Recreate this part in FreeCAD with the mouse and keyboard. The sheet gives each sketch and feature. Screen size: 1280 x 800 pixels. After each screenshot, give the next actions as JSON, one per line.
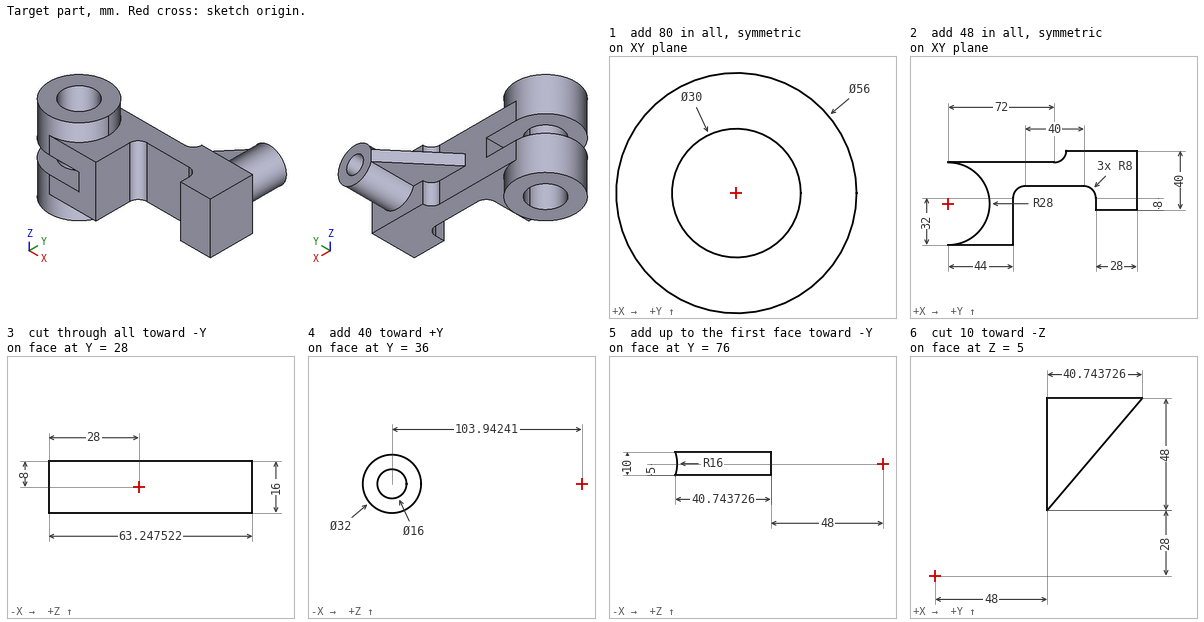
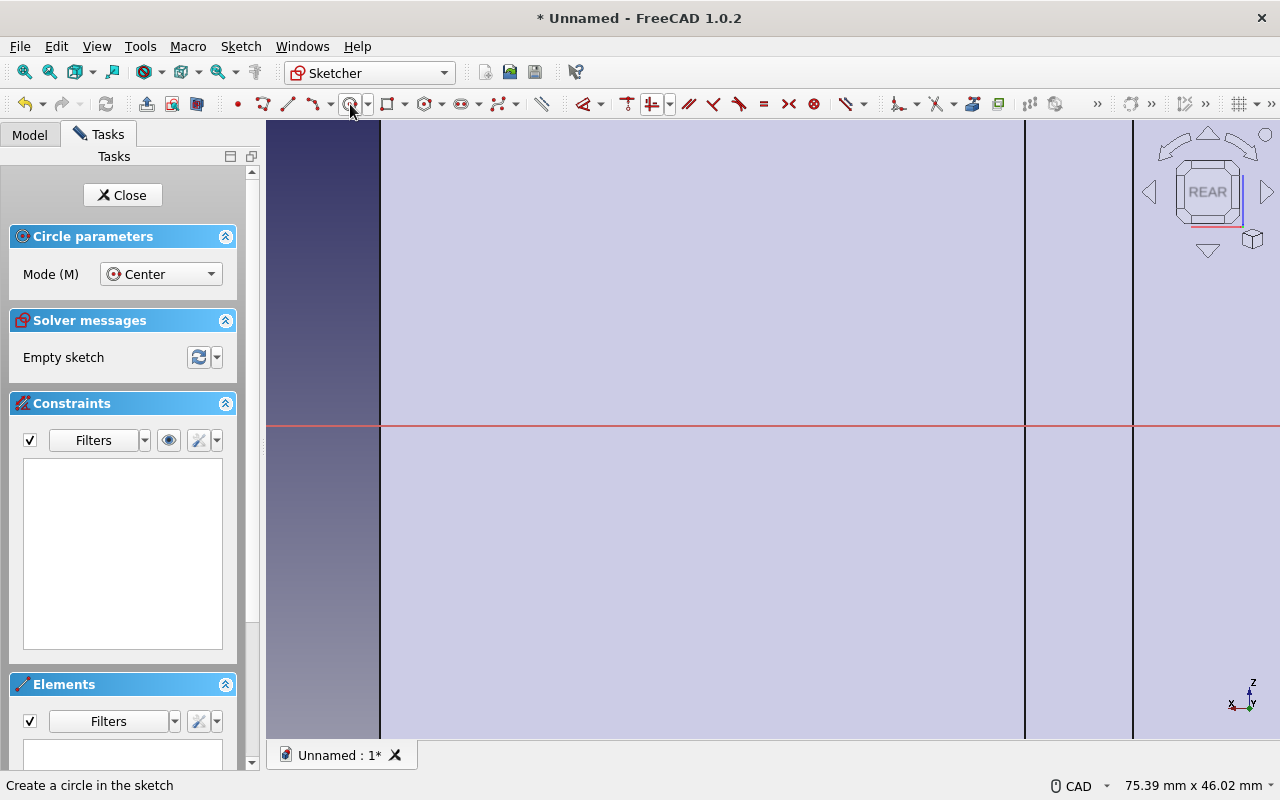
{"action": "left_click", "coordinate": [703, 426]}
{"action": "mouse_move", "coordinate": [856, 274]}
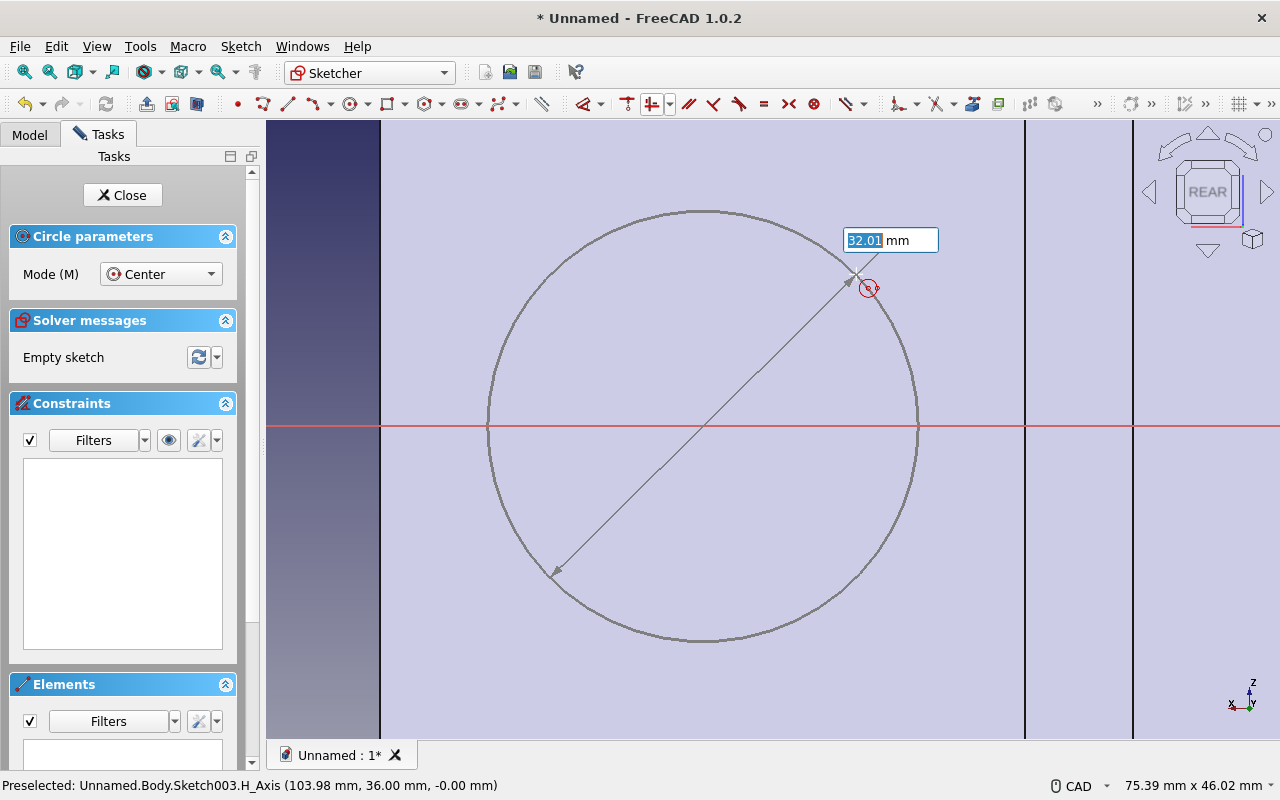
{"action": "type", "text": "32"}
{"action": "key", "text": "Return"}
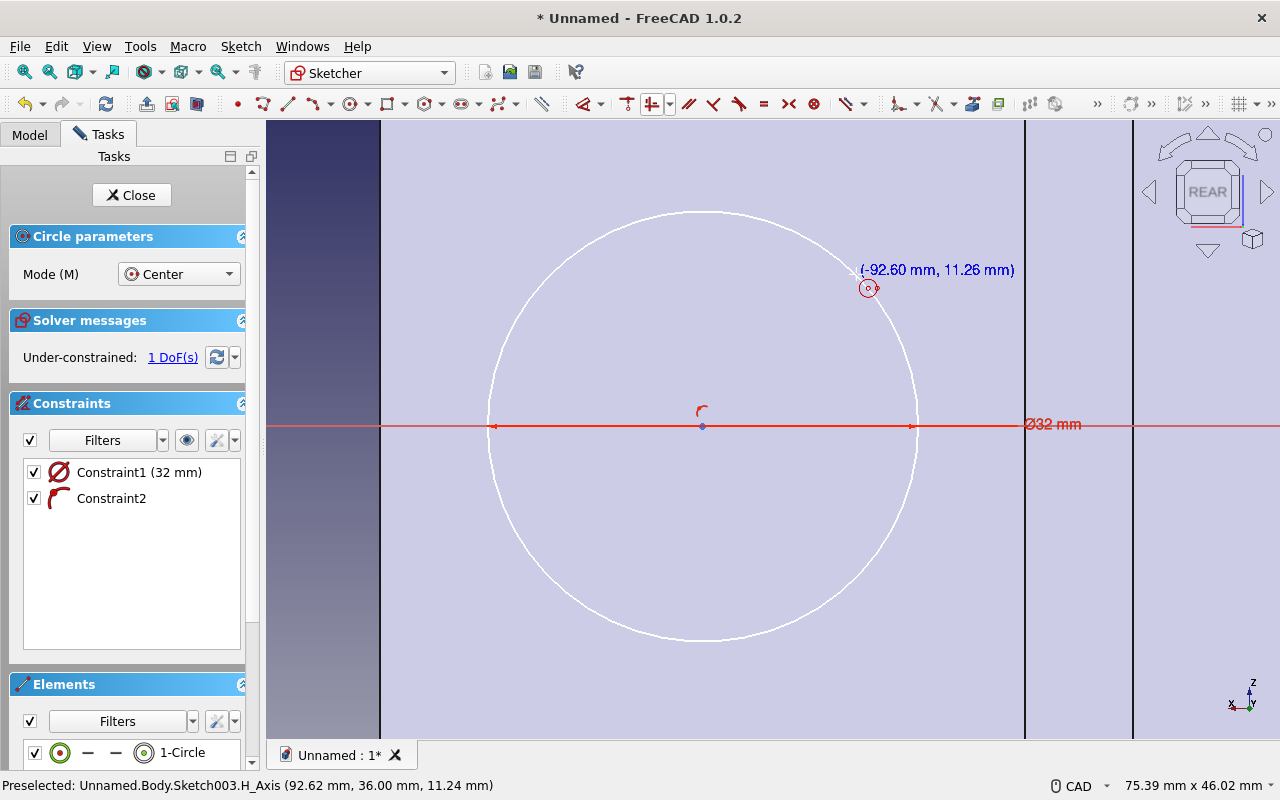
{"action": "left_click", "coordinate": [703, 426]}
{"action": "mouse_move", "coordinate": [780, 350]}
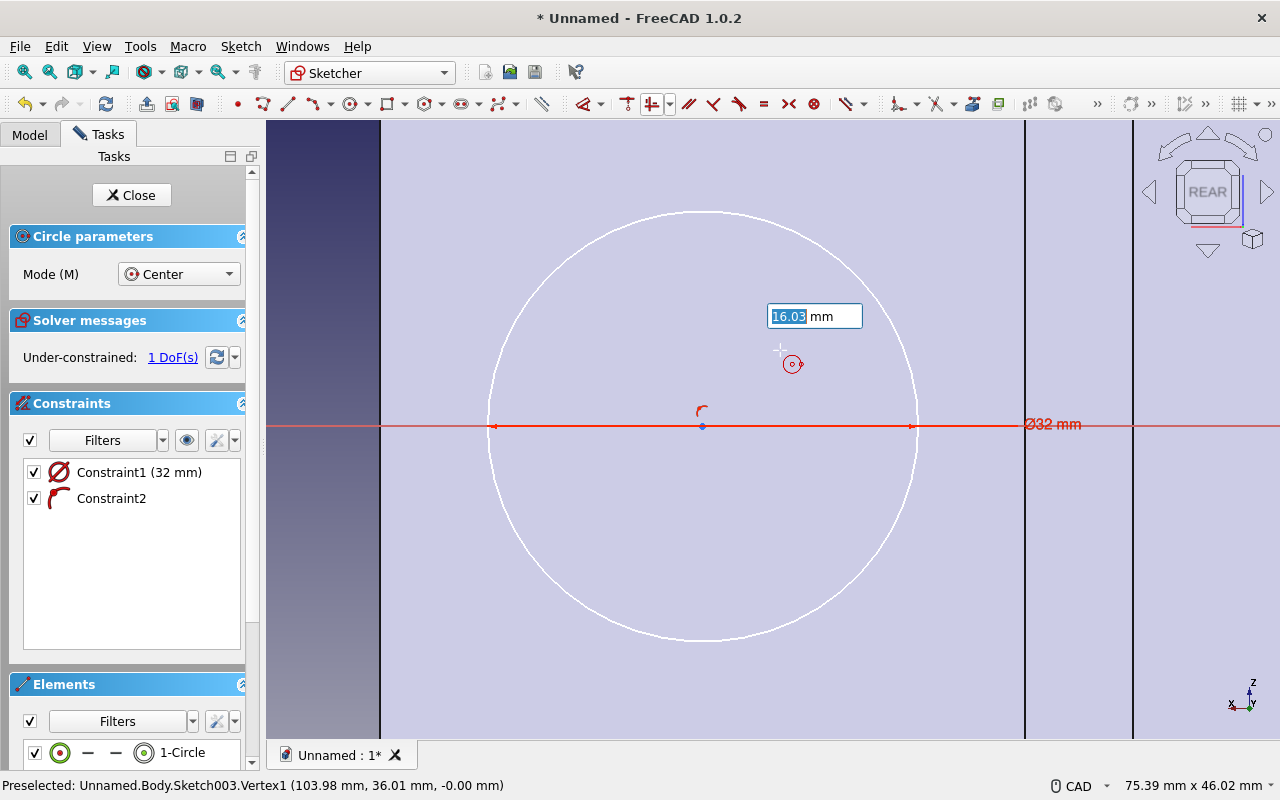
{"action": "type", "text": "16"}
{"action": "key", "text": "Return"}
{"action": "key", "text": "Escape"}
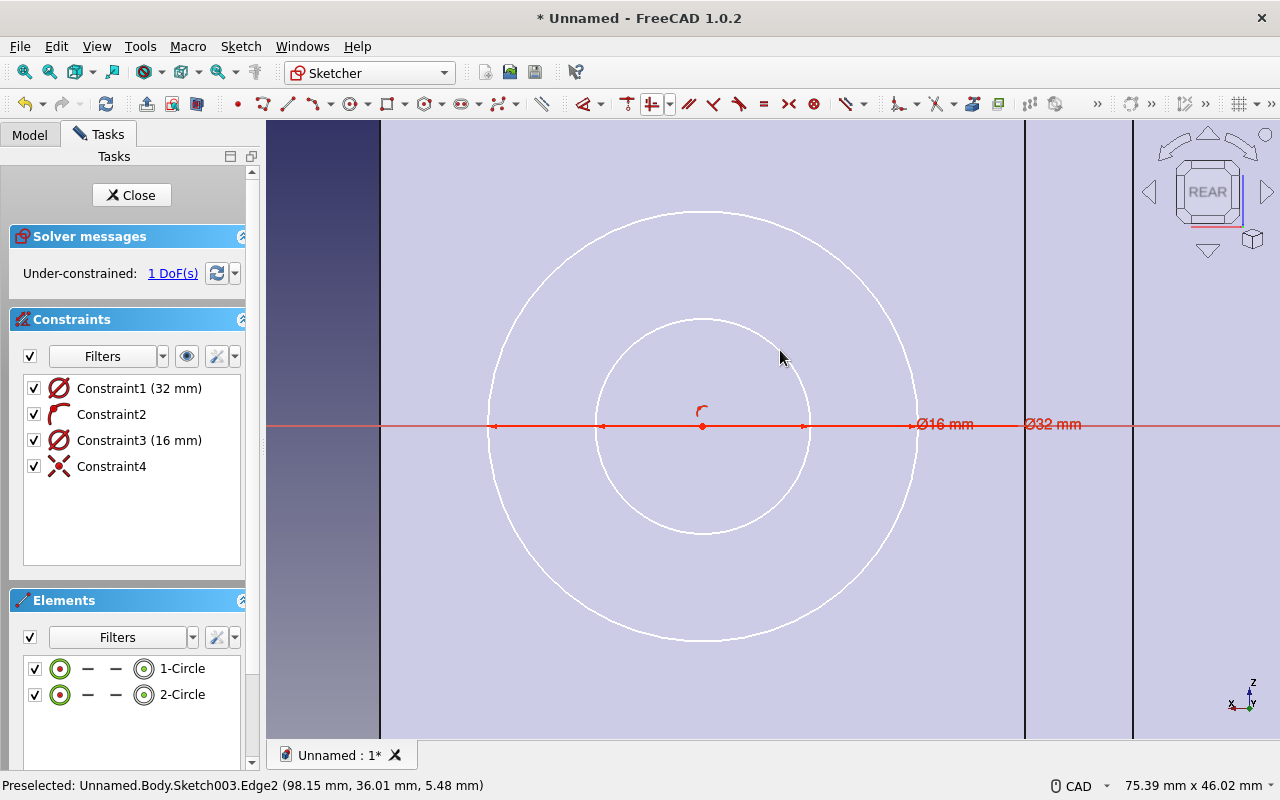
{"action": "left_click", "coordinate": [582, 104]}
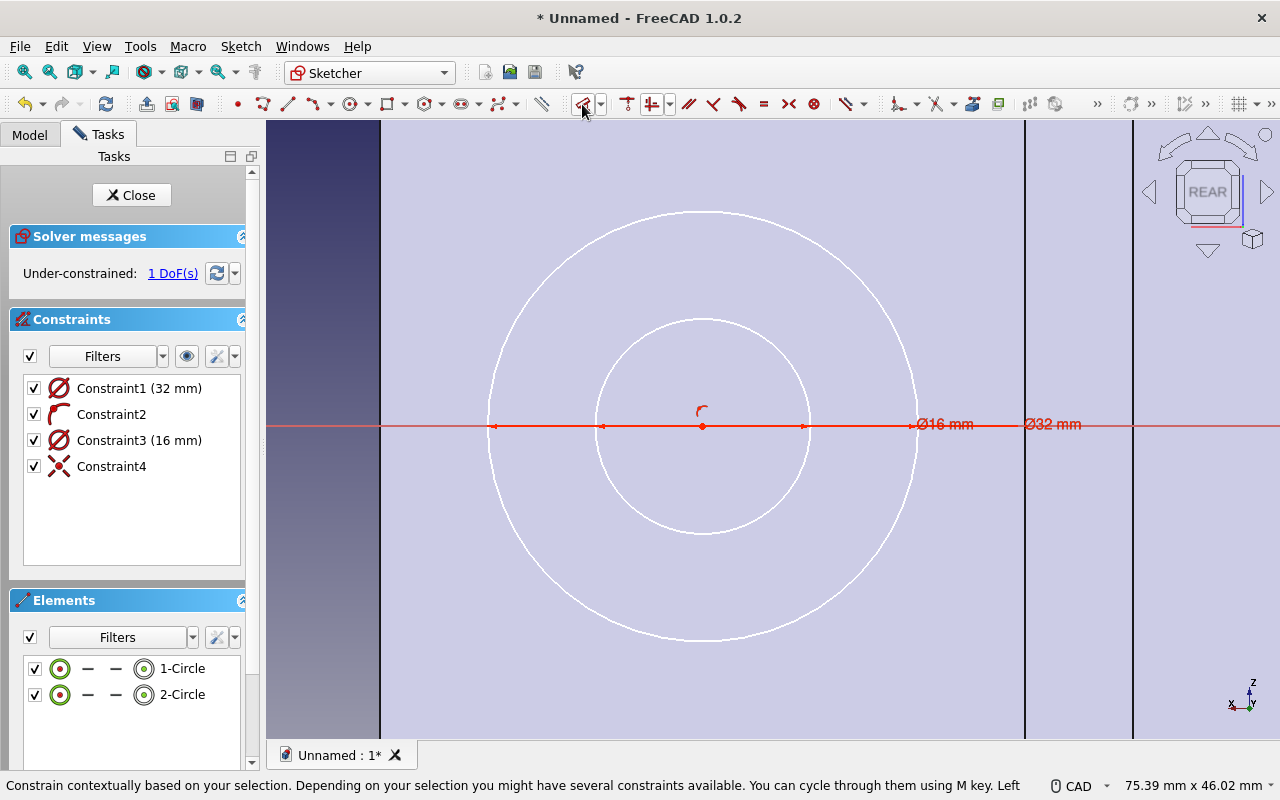
{"action": "left_click", "coordinate": [703, 426]}
{"action": "left_click", "coordinate": [1004, 460]}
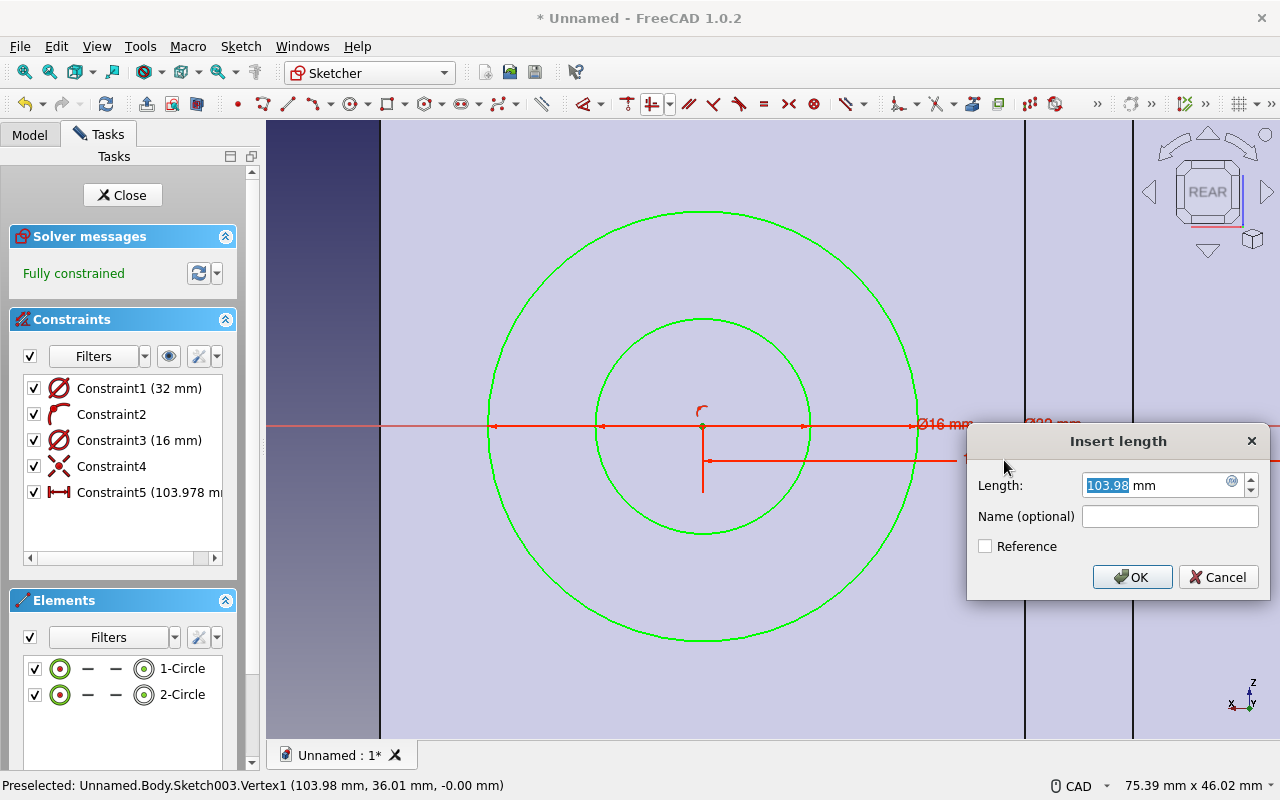
{"action": "type", "text": "103.94241"}
{"action": "key", "text": "Return"}
{"action": "key", "text": "Escape"}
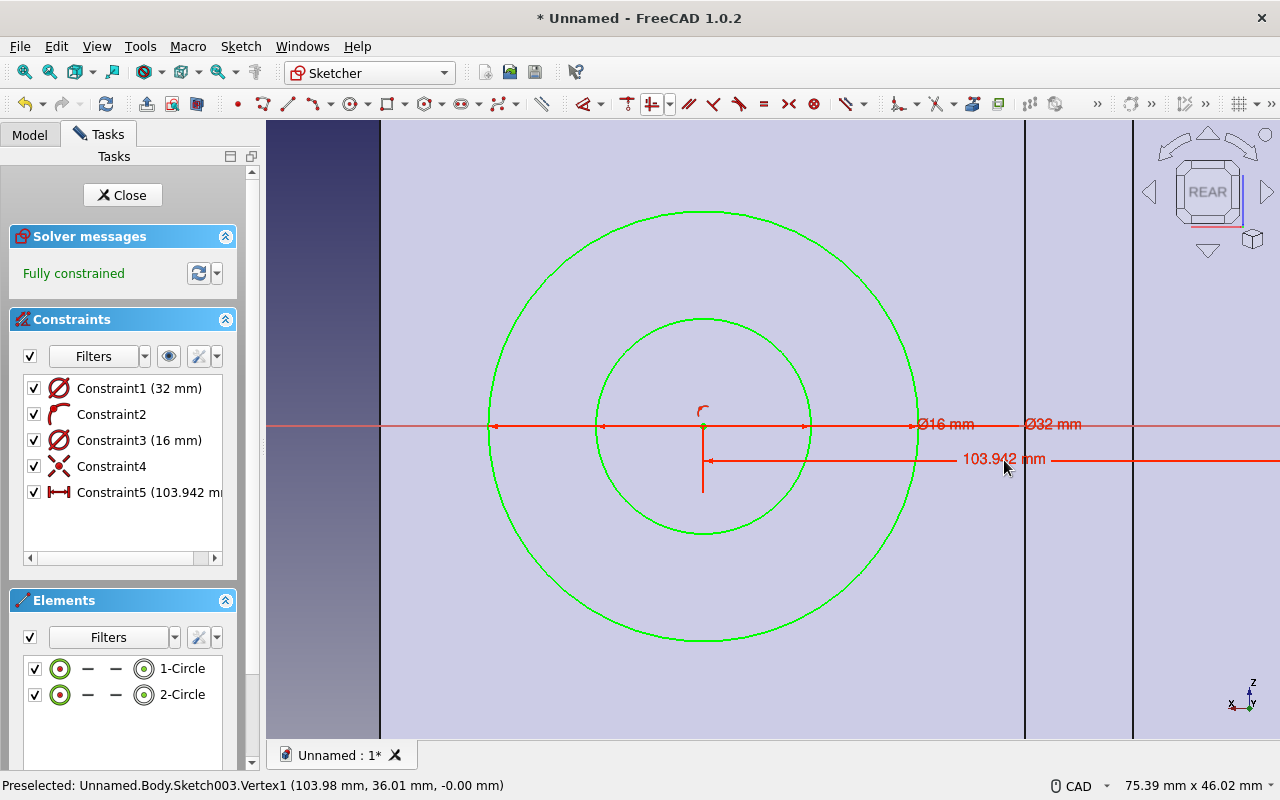
{"action": "left_click", "coordinate": [123, 195]}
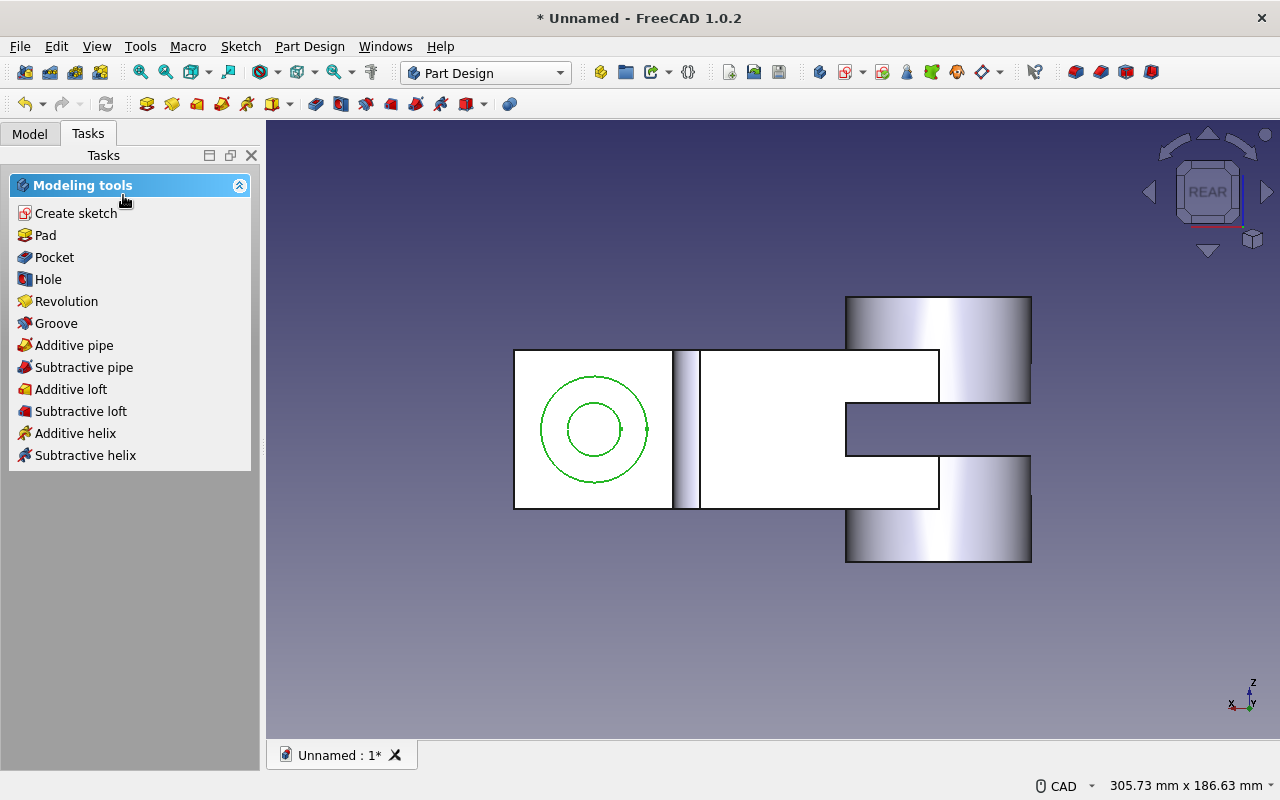
{"action": "left_click", "coordinate": [147, 104]}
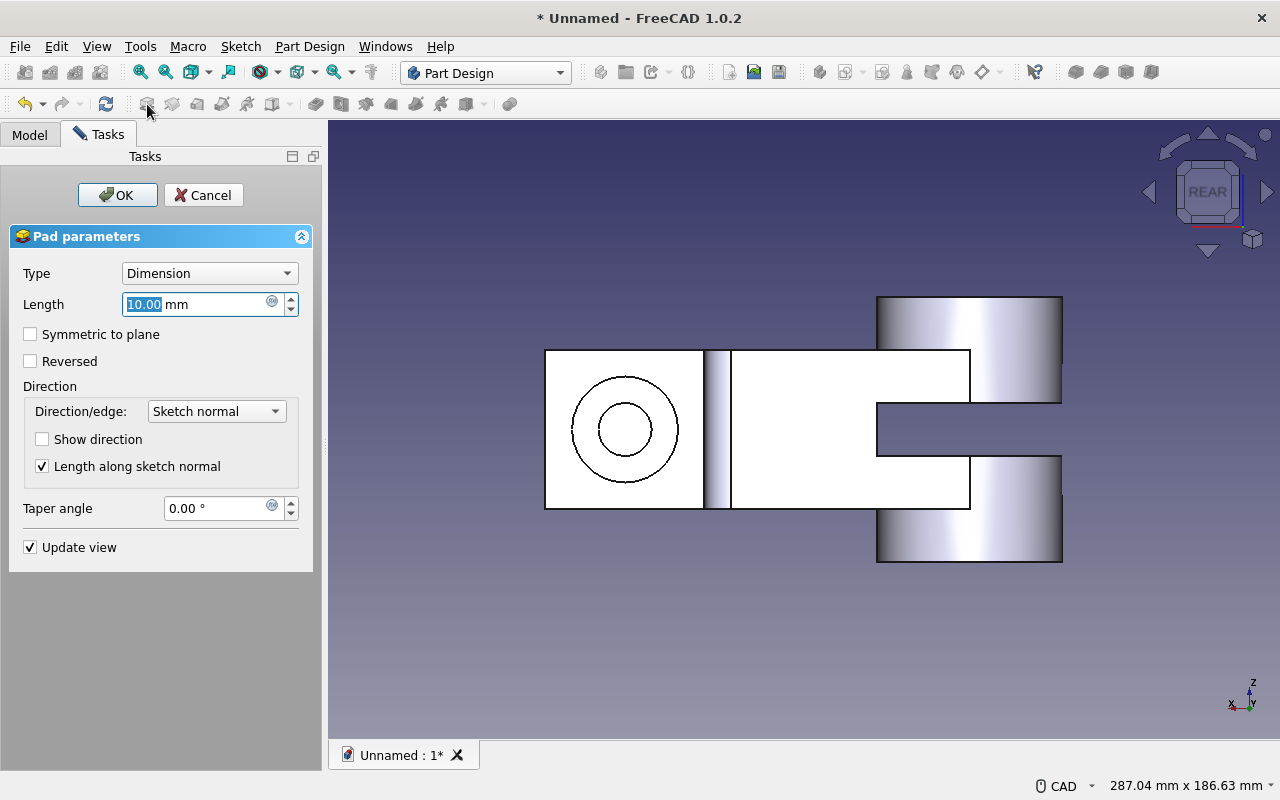
{"action": "type", "text": "40"}
{"action": "key", "text": "Tab"}